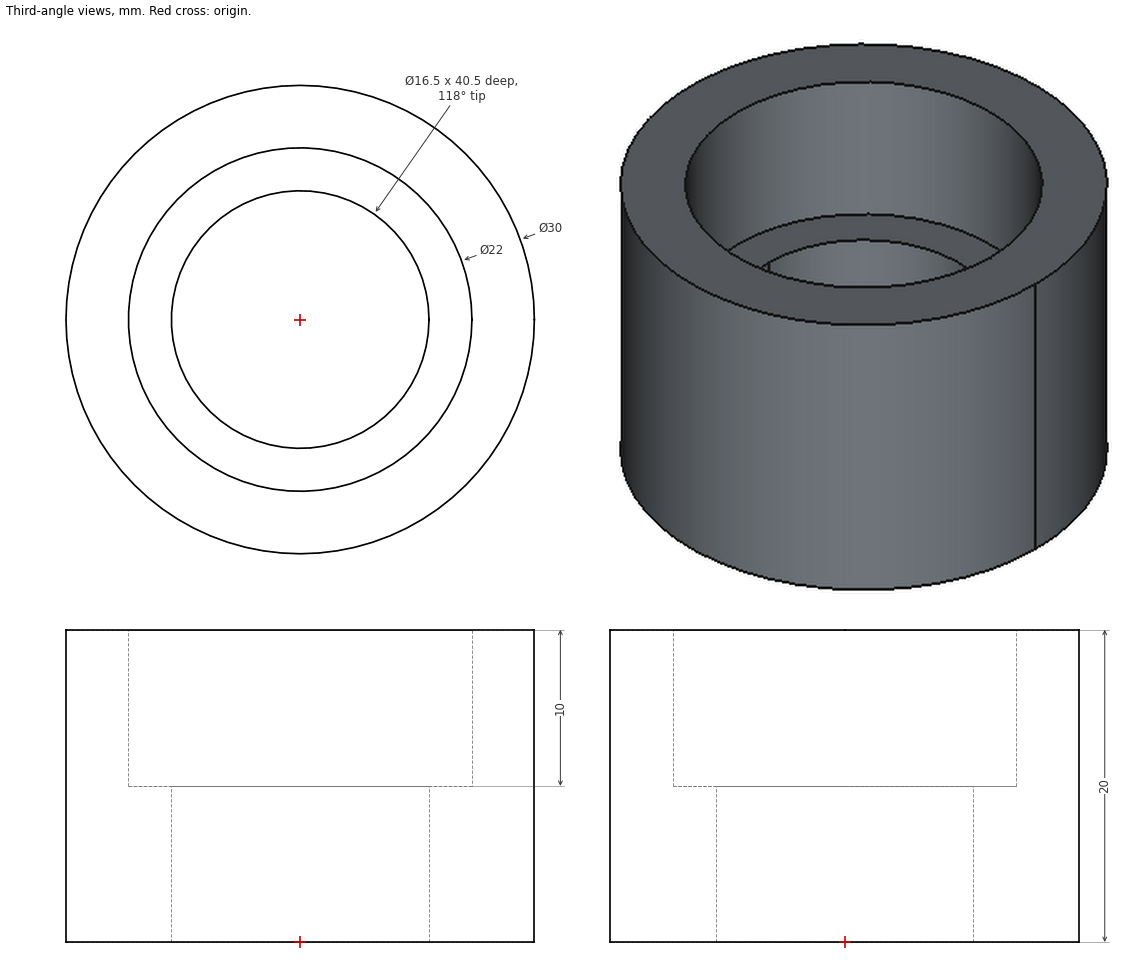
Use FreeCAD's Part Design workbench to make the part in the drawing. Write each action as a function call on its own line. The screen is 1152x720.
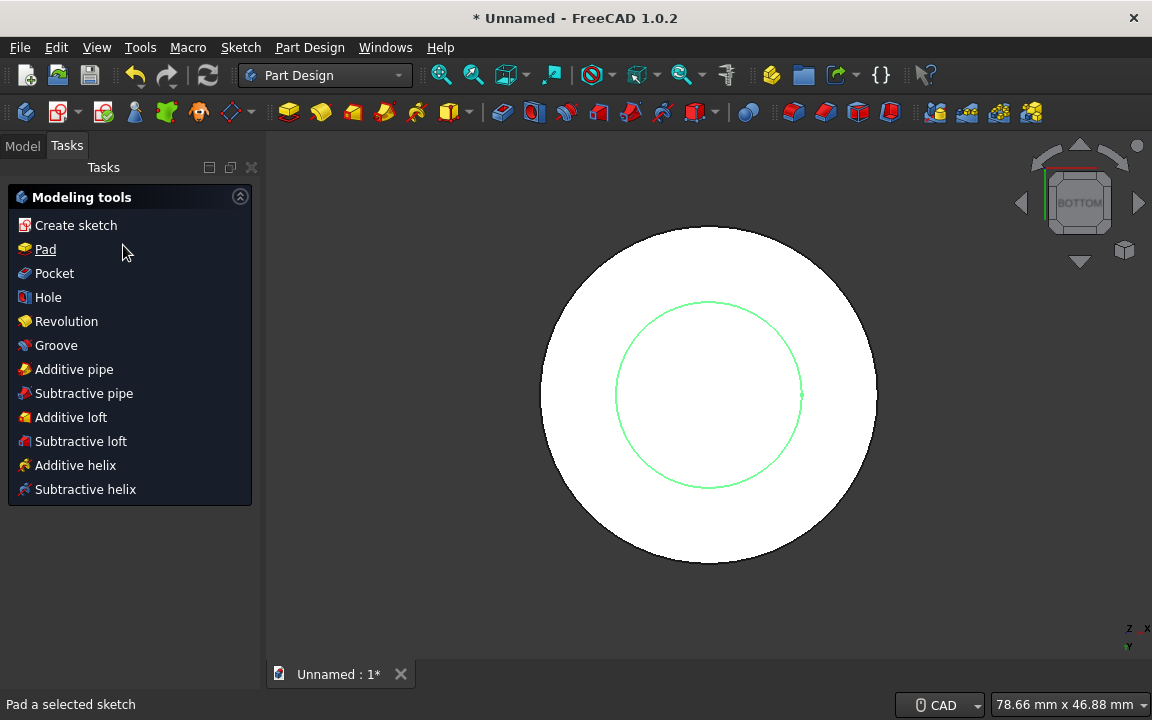
click(536, 112)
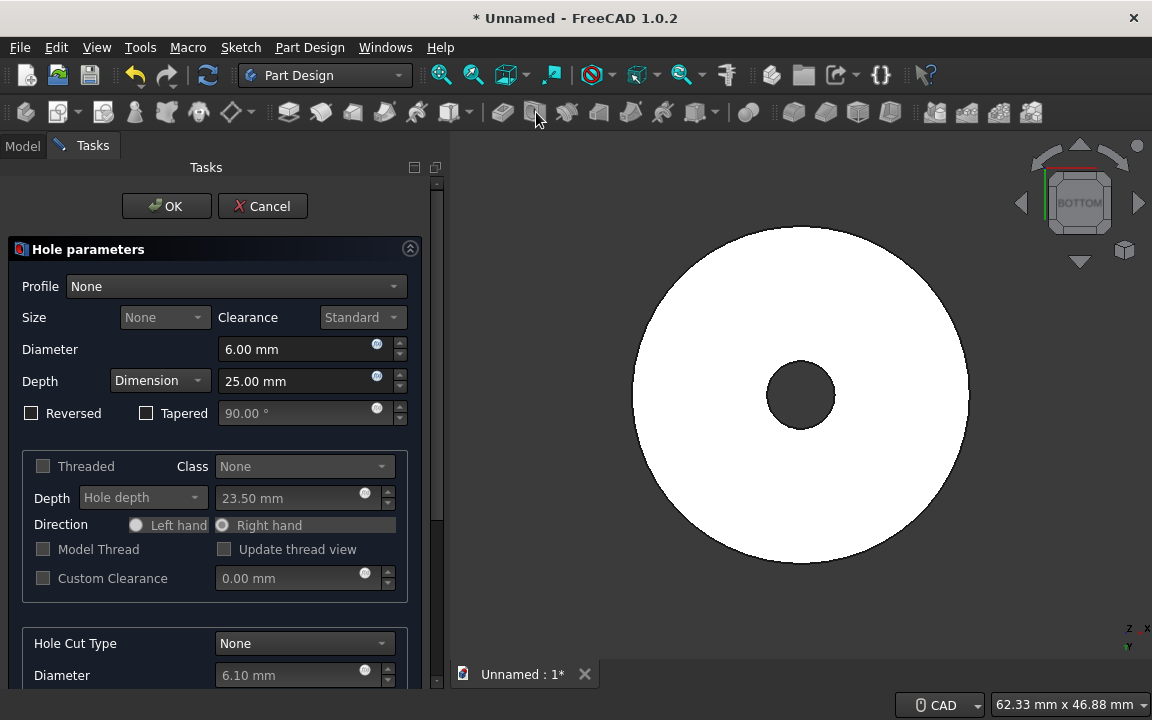
triple_click(305, 349)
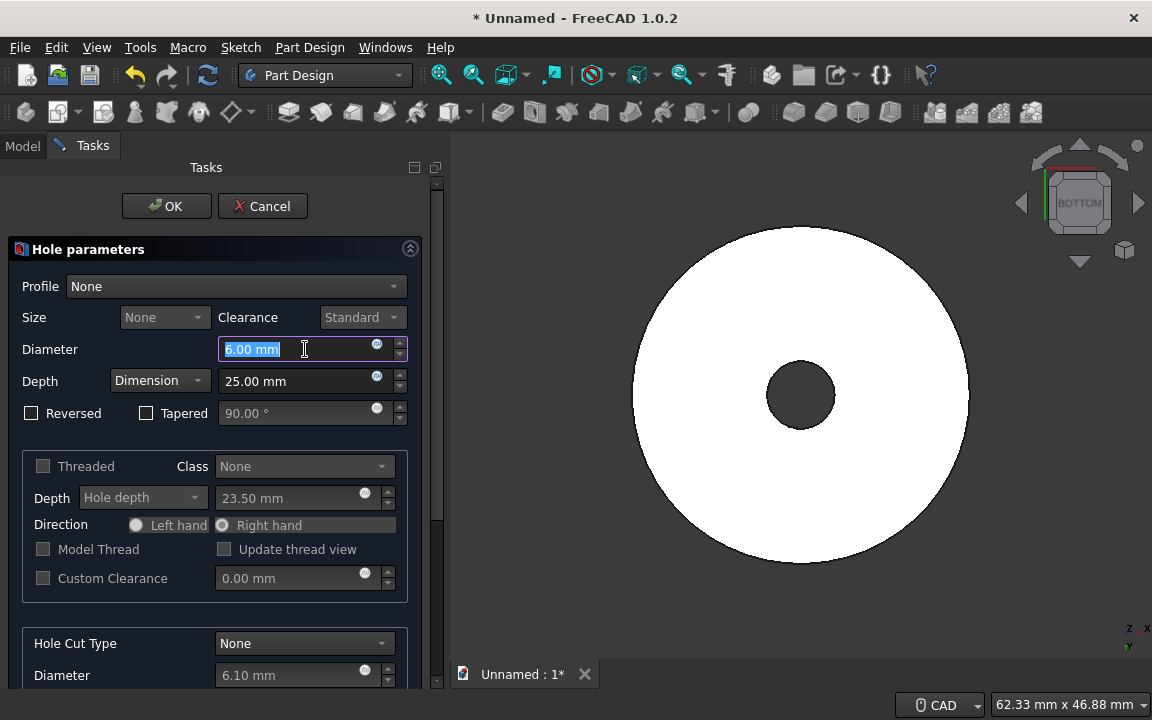
text(16.5)
key(Tab)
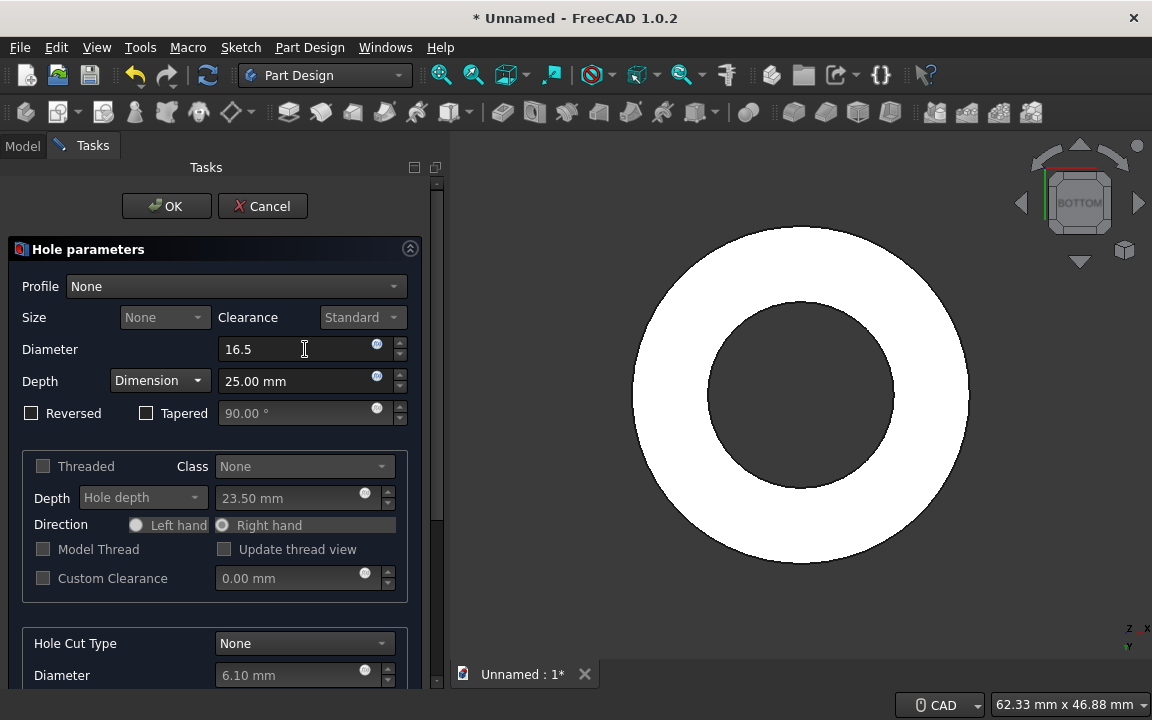
triple_click(305, 381)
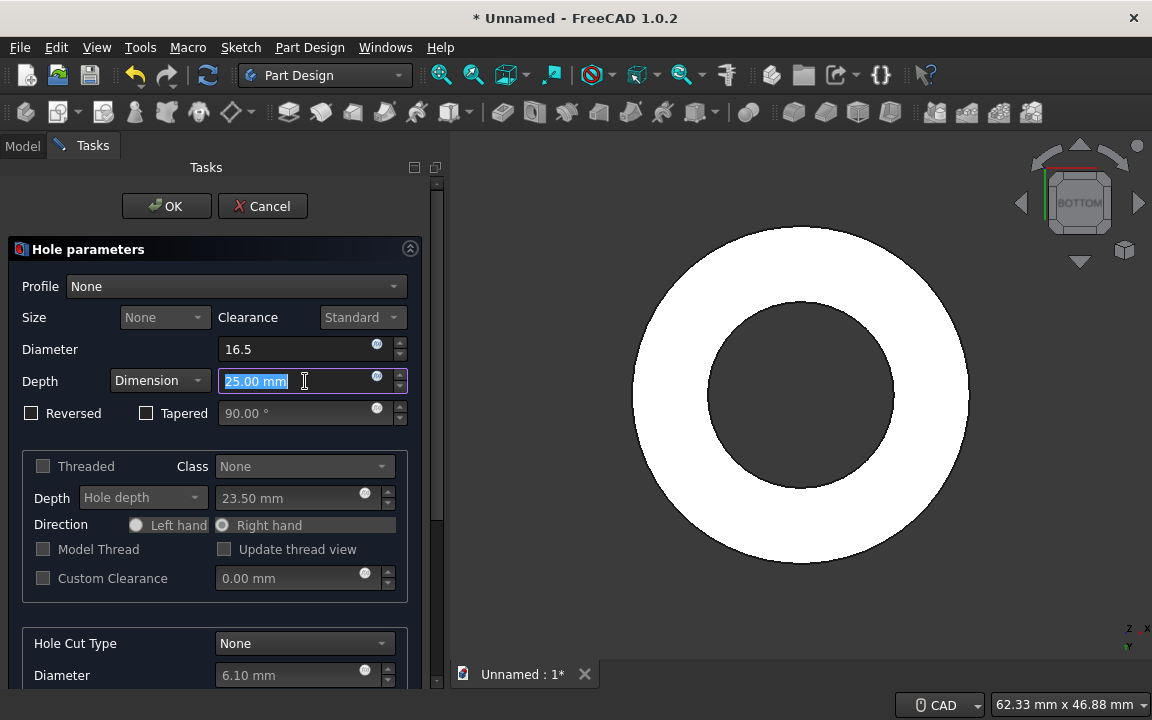
text(40.5)
key(Tab)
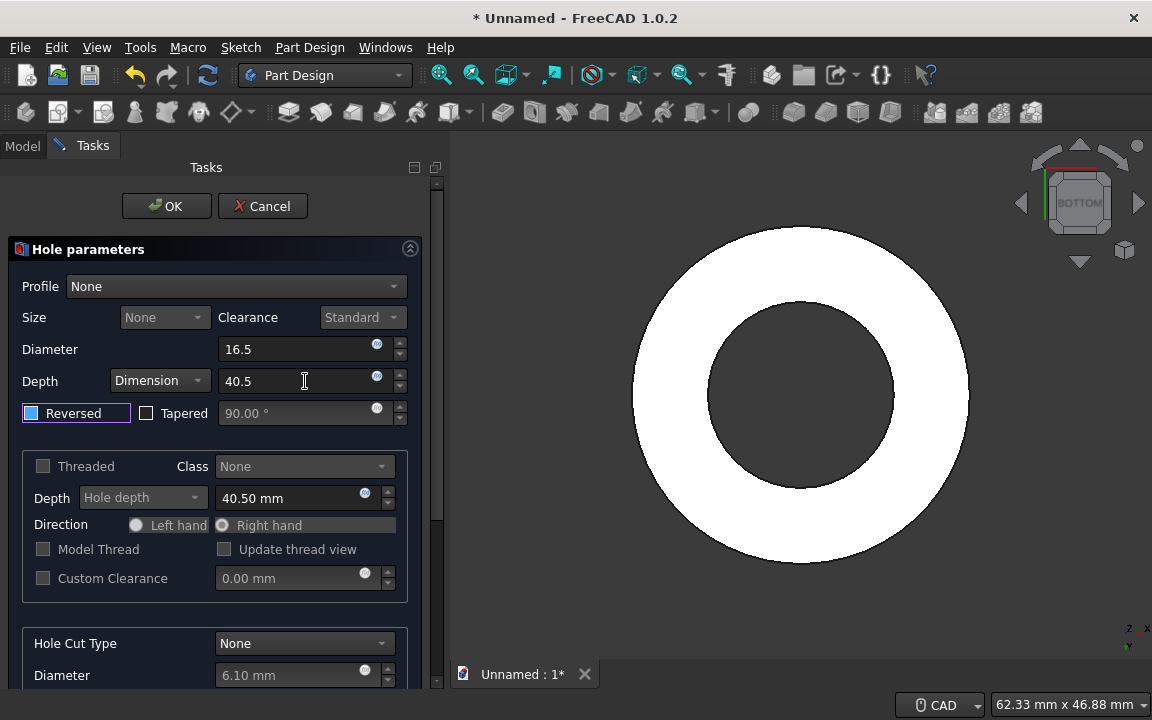
click(167, 206)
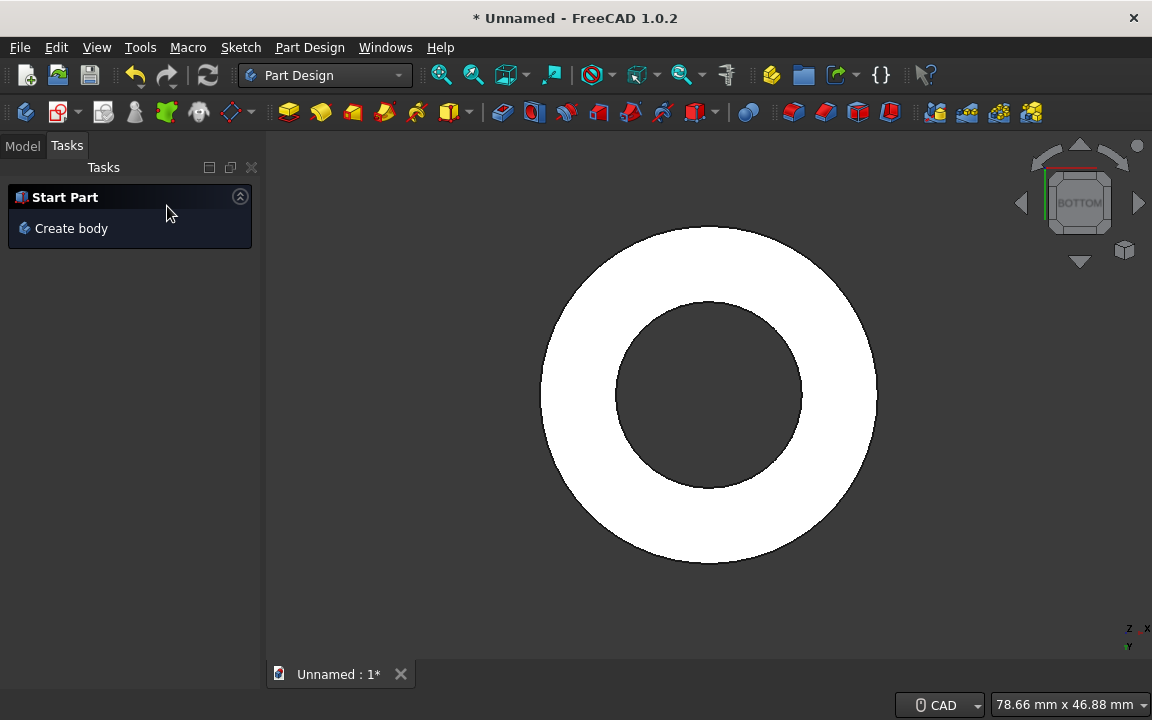
key(0)